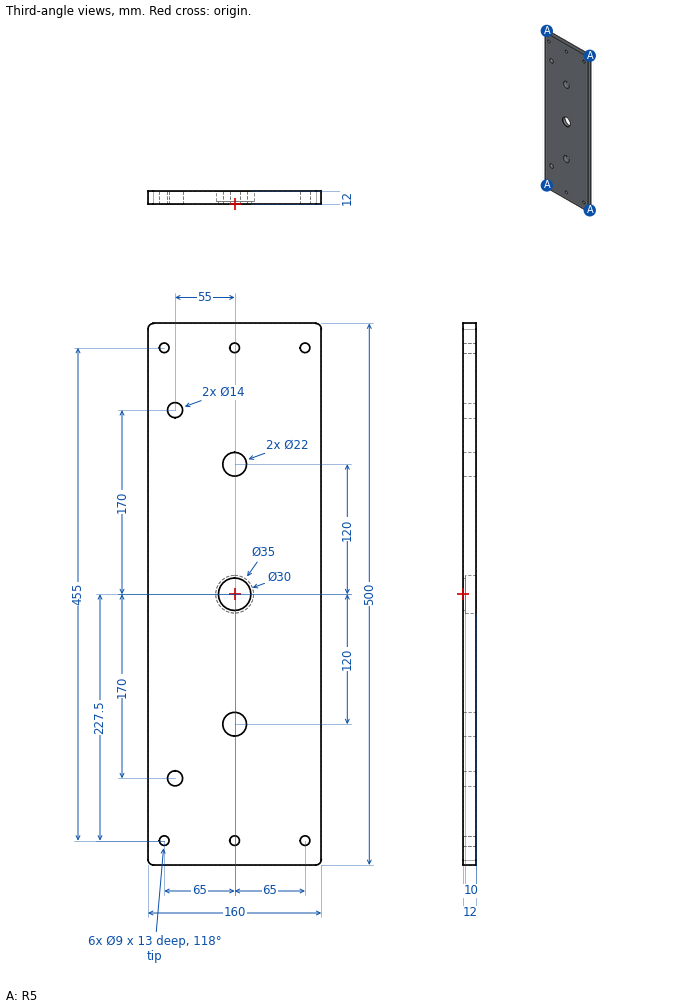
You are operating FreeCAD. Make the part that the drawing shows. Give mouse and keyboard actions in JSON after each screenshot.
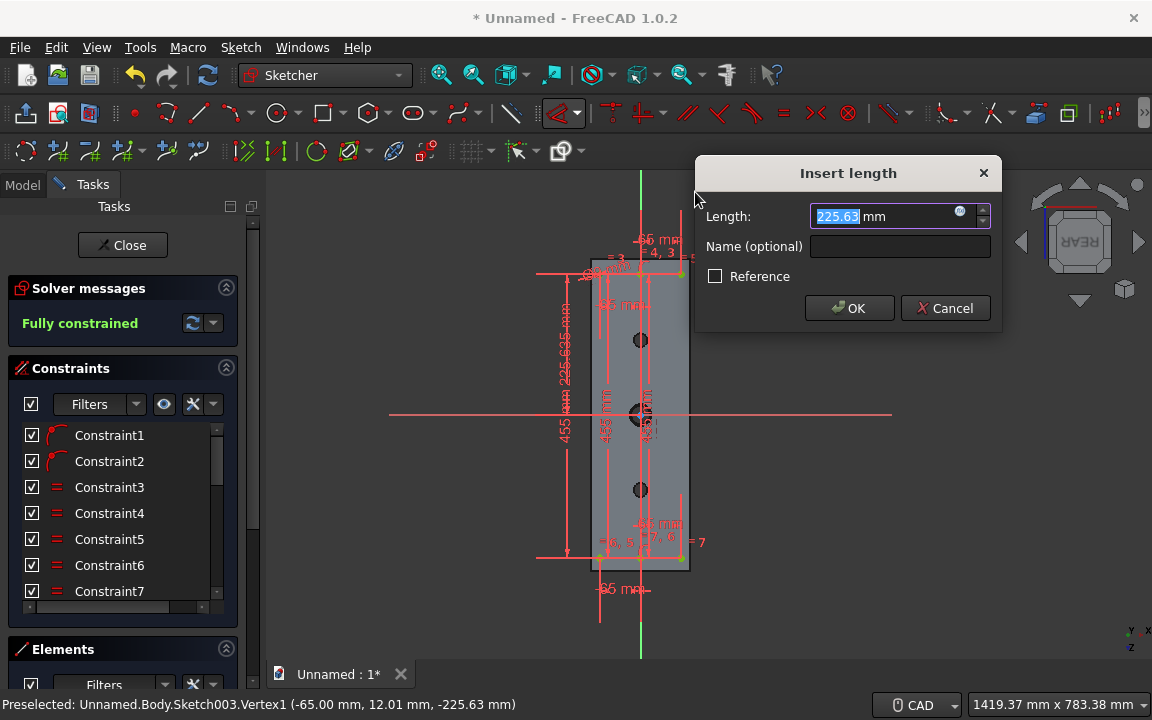
{"action": "type", "text": "227.5"}
{"action": "key", "text": "Return"}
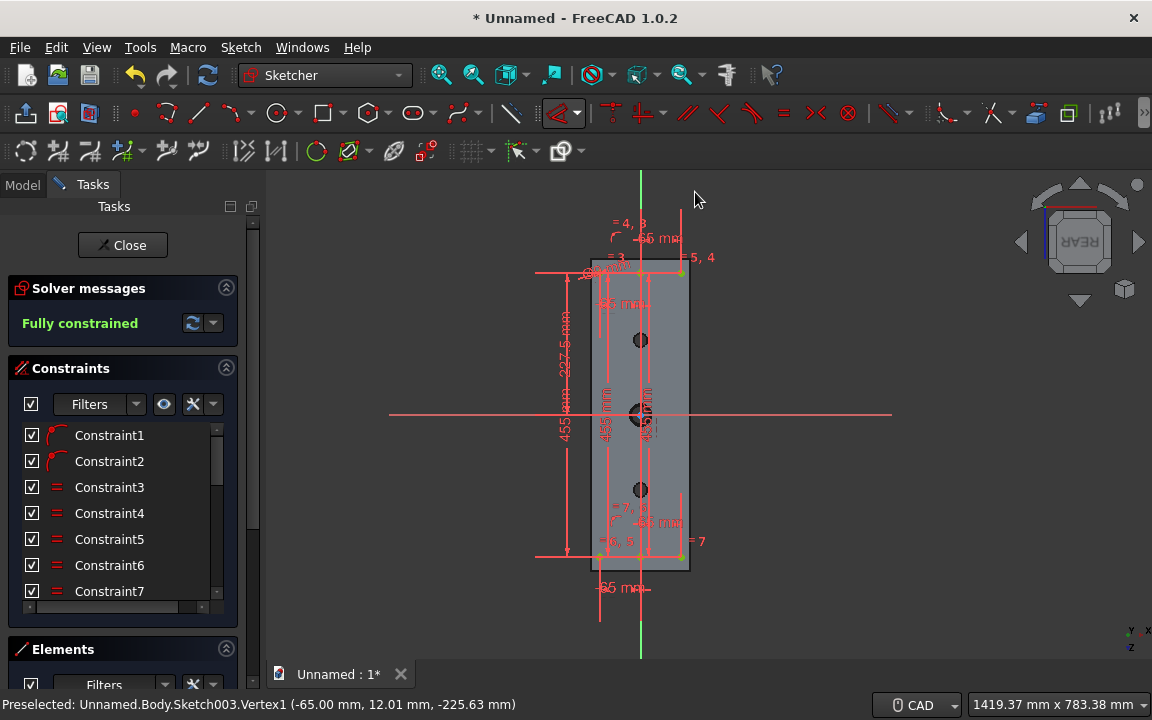
{"action": "left_click", "coordinate": [123, 245]}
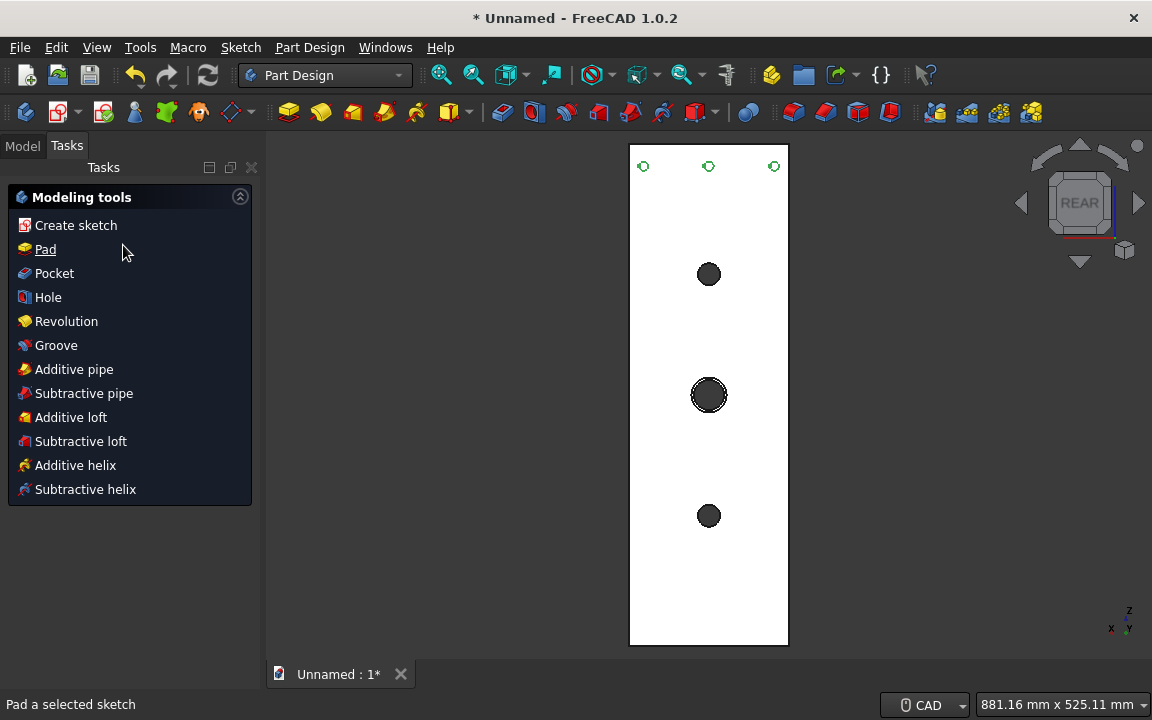
{"action": "left_click", "coordinate": [536, 112]}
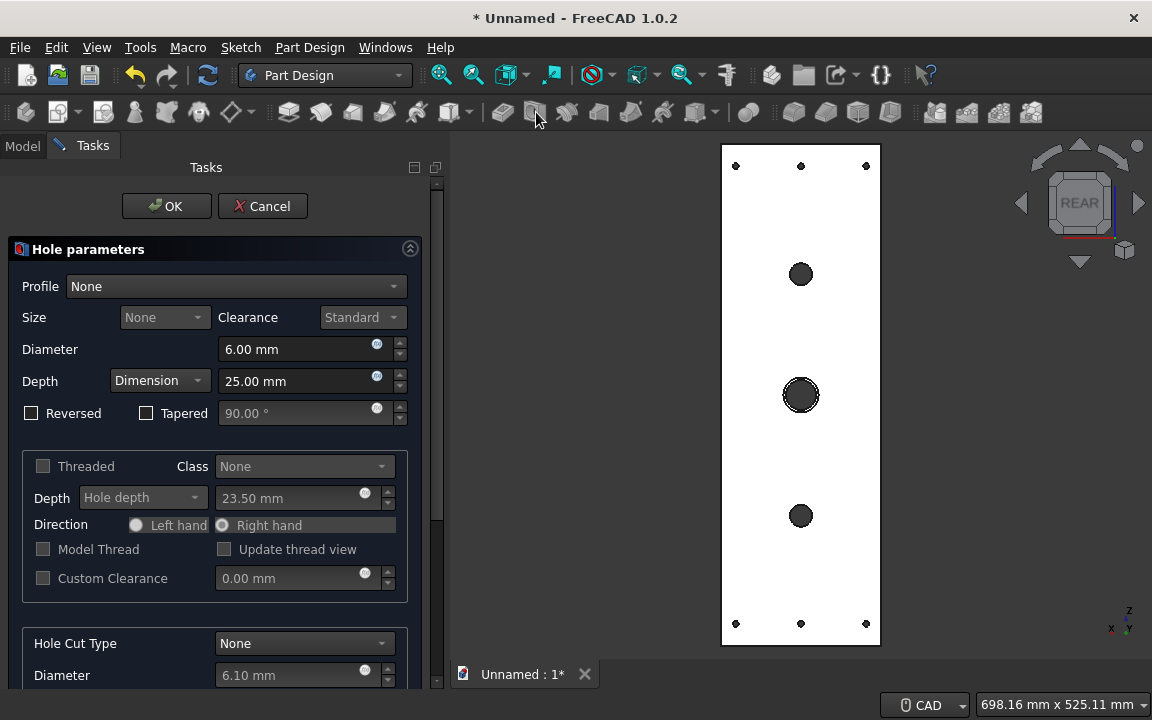
{"action": "triple_click", "coordinate": [305, 349]}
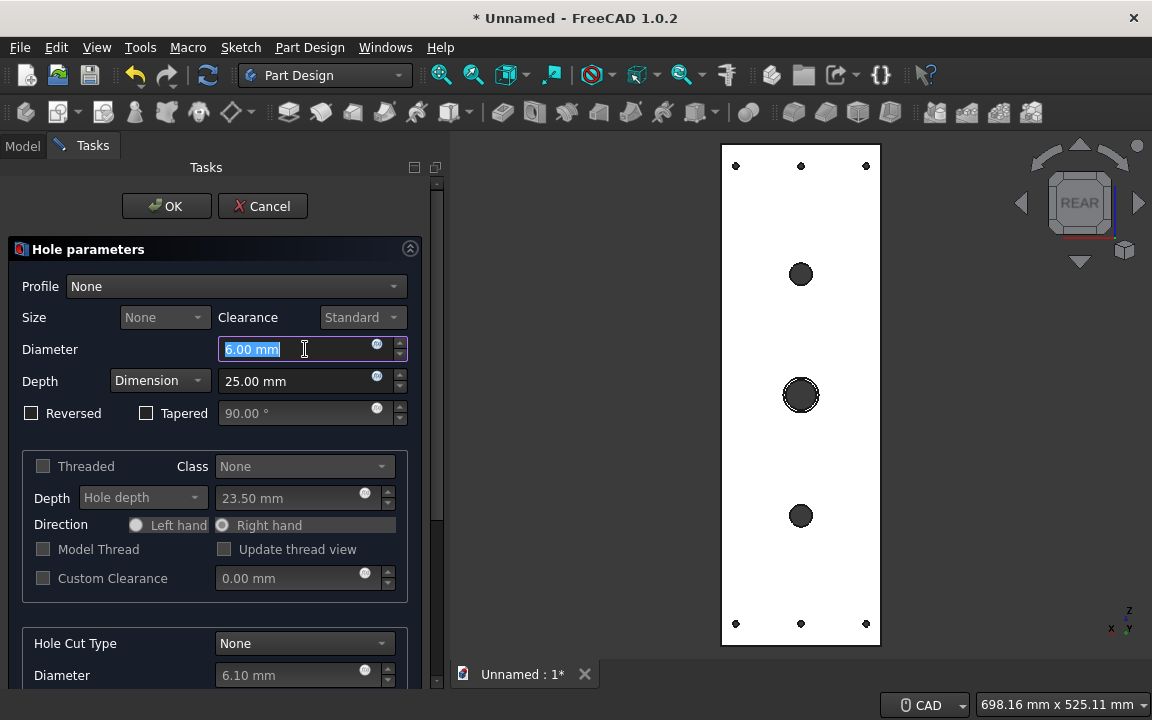
{"action": "type", "text": "9"}
{"action": "key", "text": "Tab"}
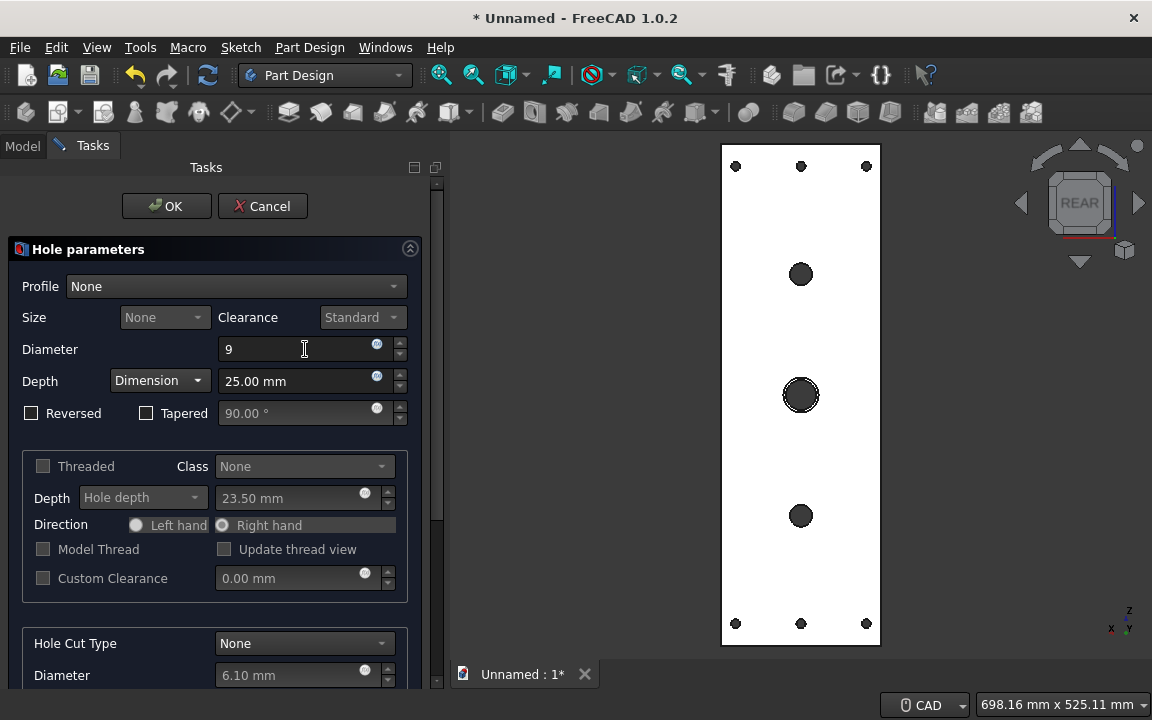
{"action": "triple_click", "coordinate": [305, 381]}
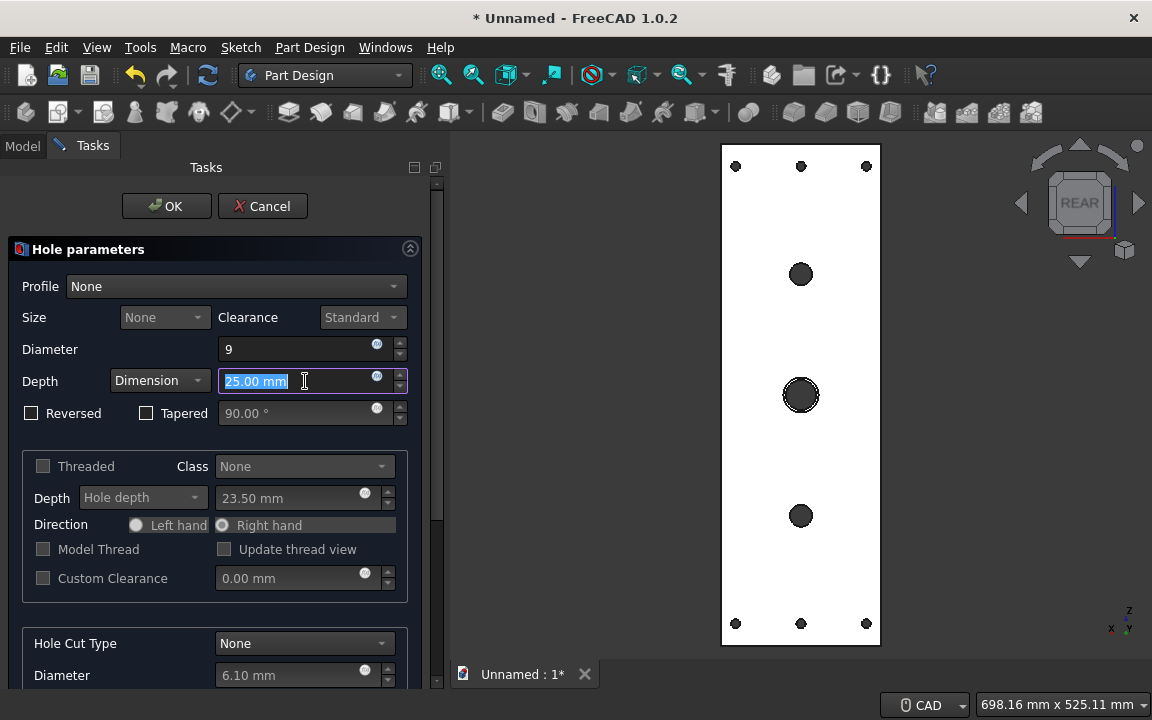
{"action": "type", "text": "13"}
{"action": "key", "text": "Tab"}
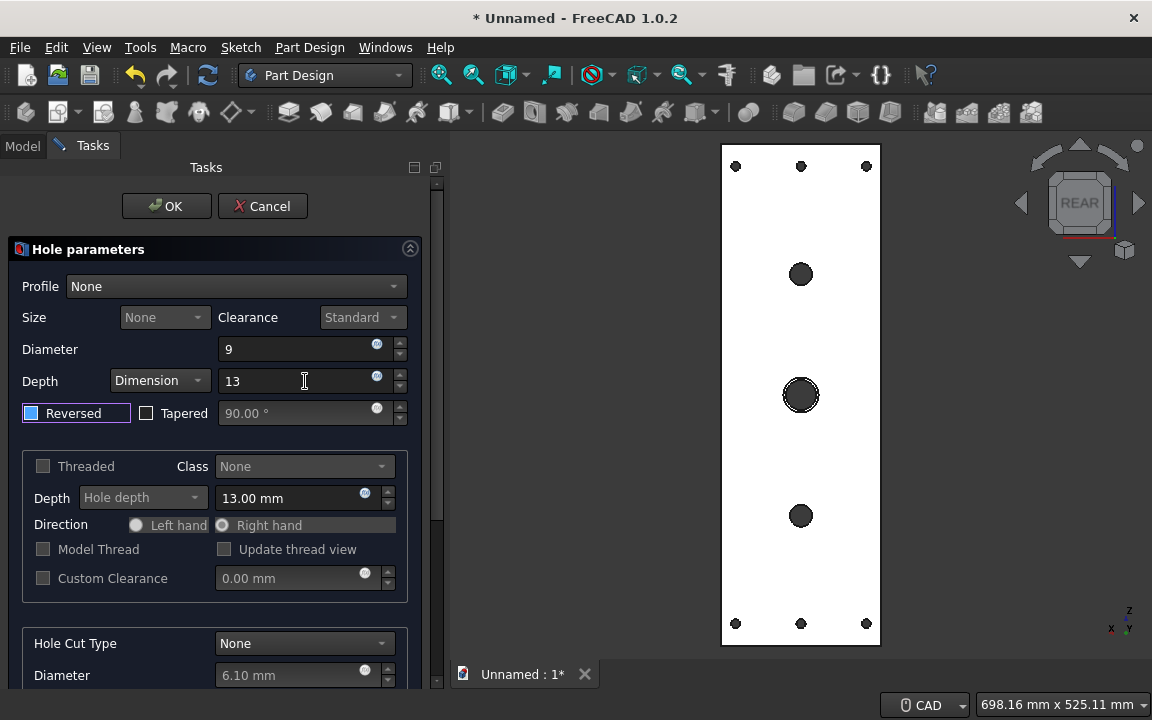
{"action": "left_click", "coordinate": [167, 206]}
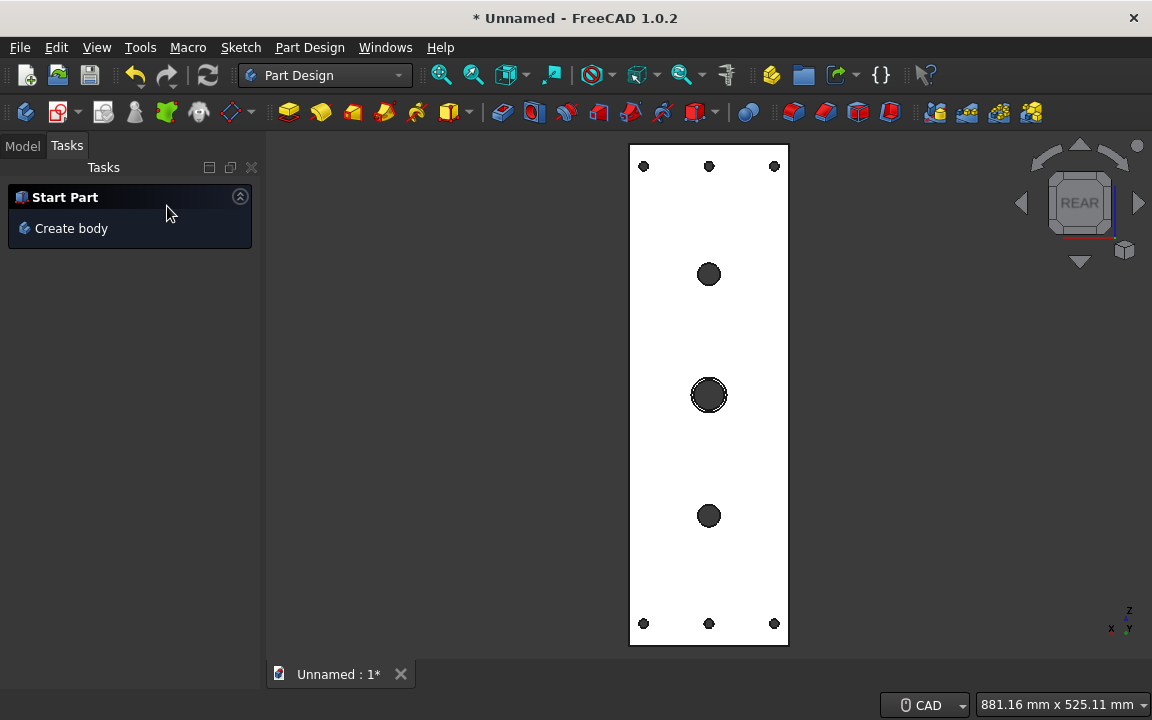
{"action": "key", "text": "0"}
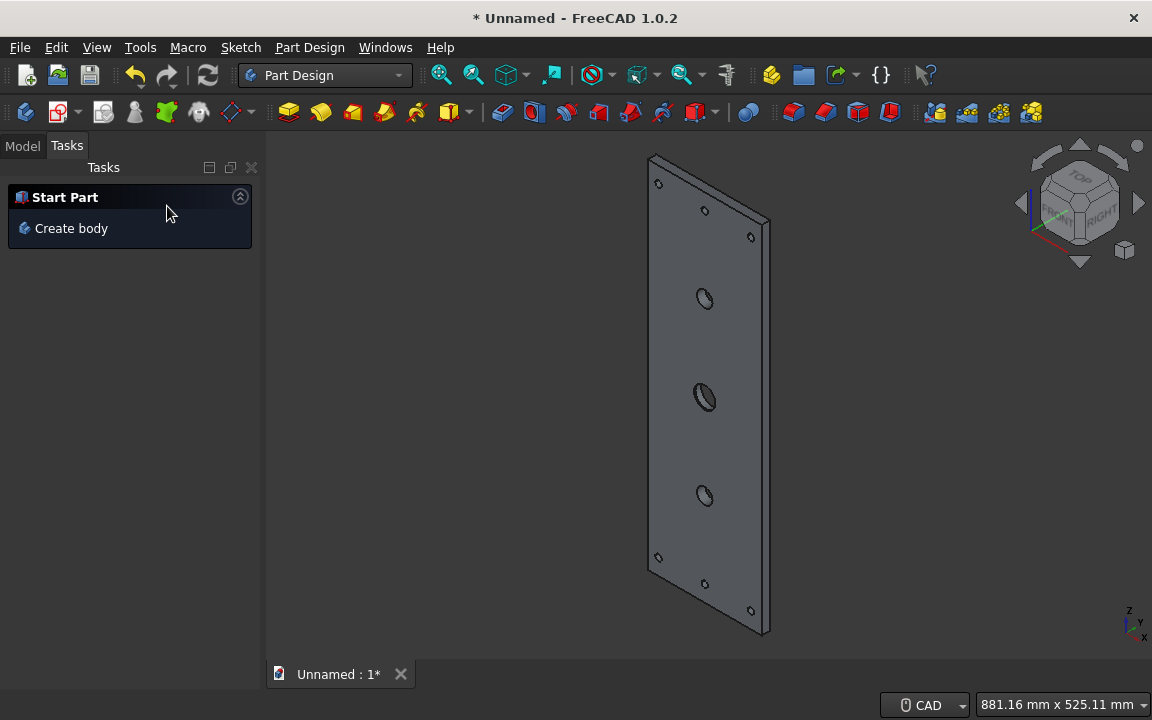
{"action": "left_click", "coordinate": [768, 221]}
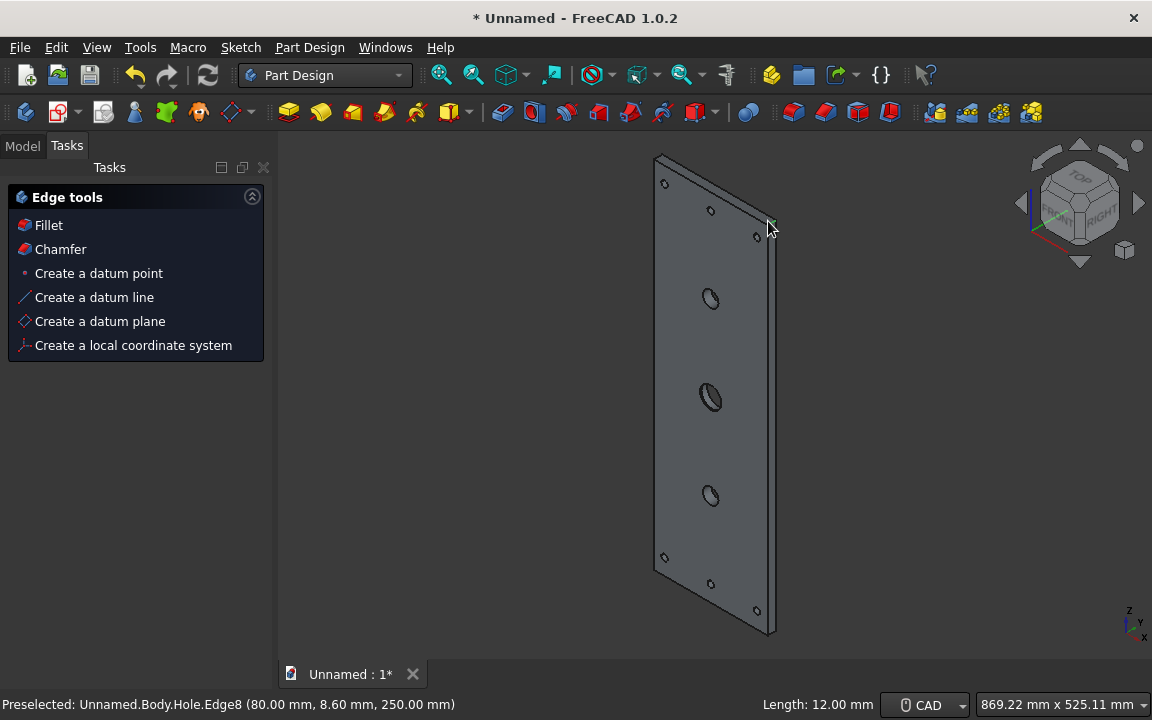
{"action": "key", "text": "2"}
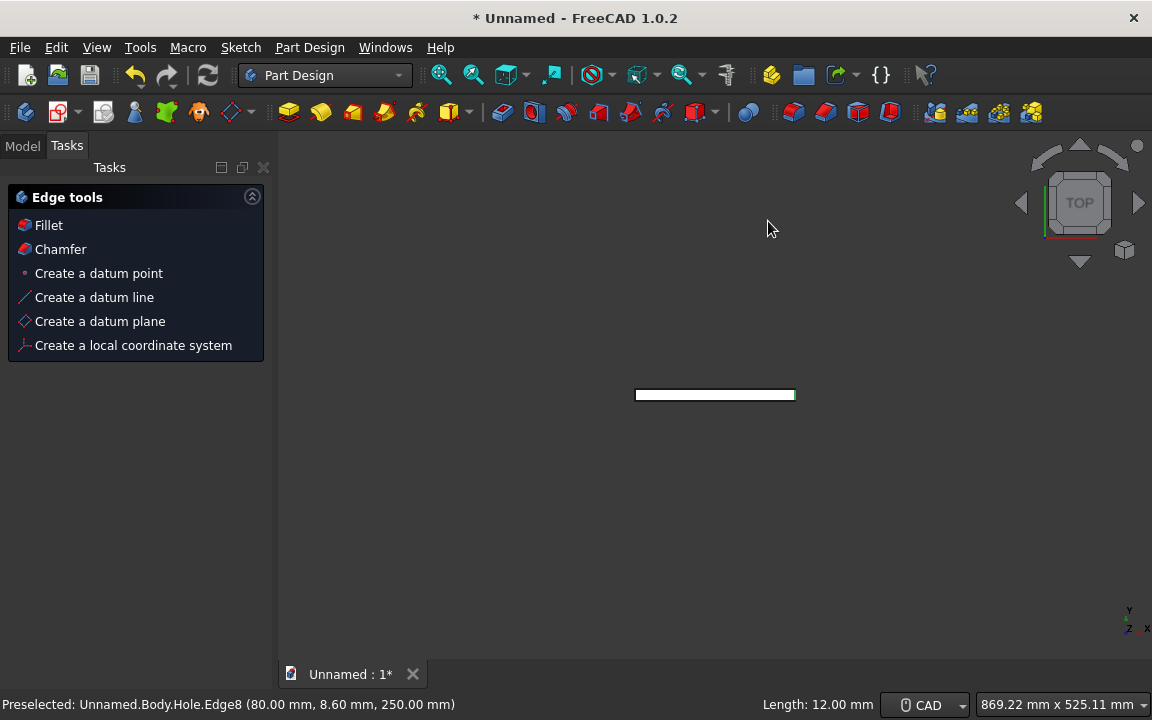
{"action": "key", "text": "v f"}